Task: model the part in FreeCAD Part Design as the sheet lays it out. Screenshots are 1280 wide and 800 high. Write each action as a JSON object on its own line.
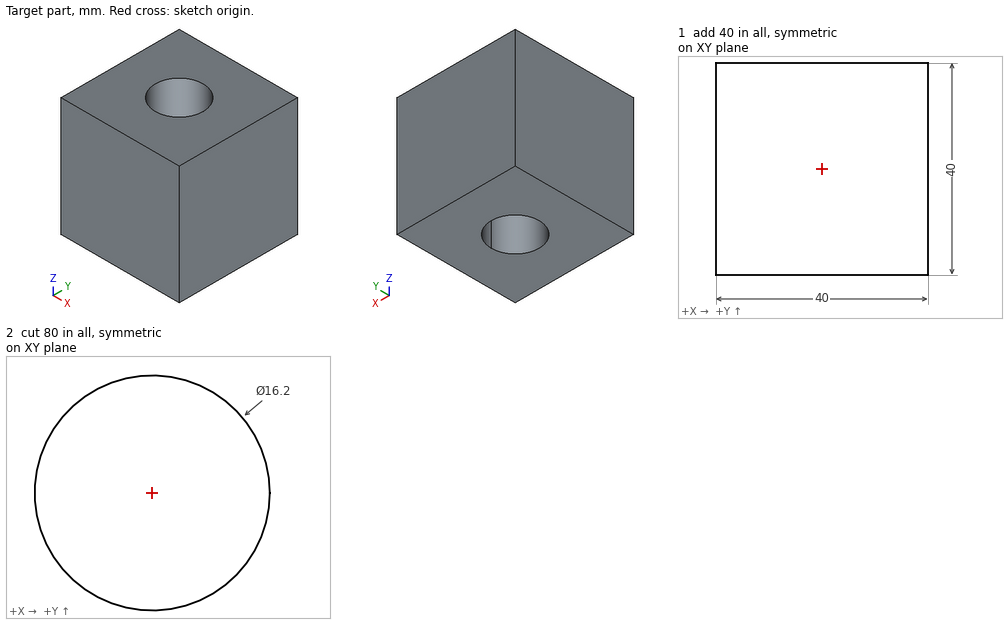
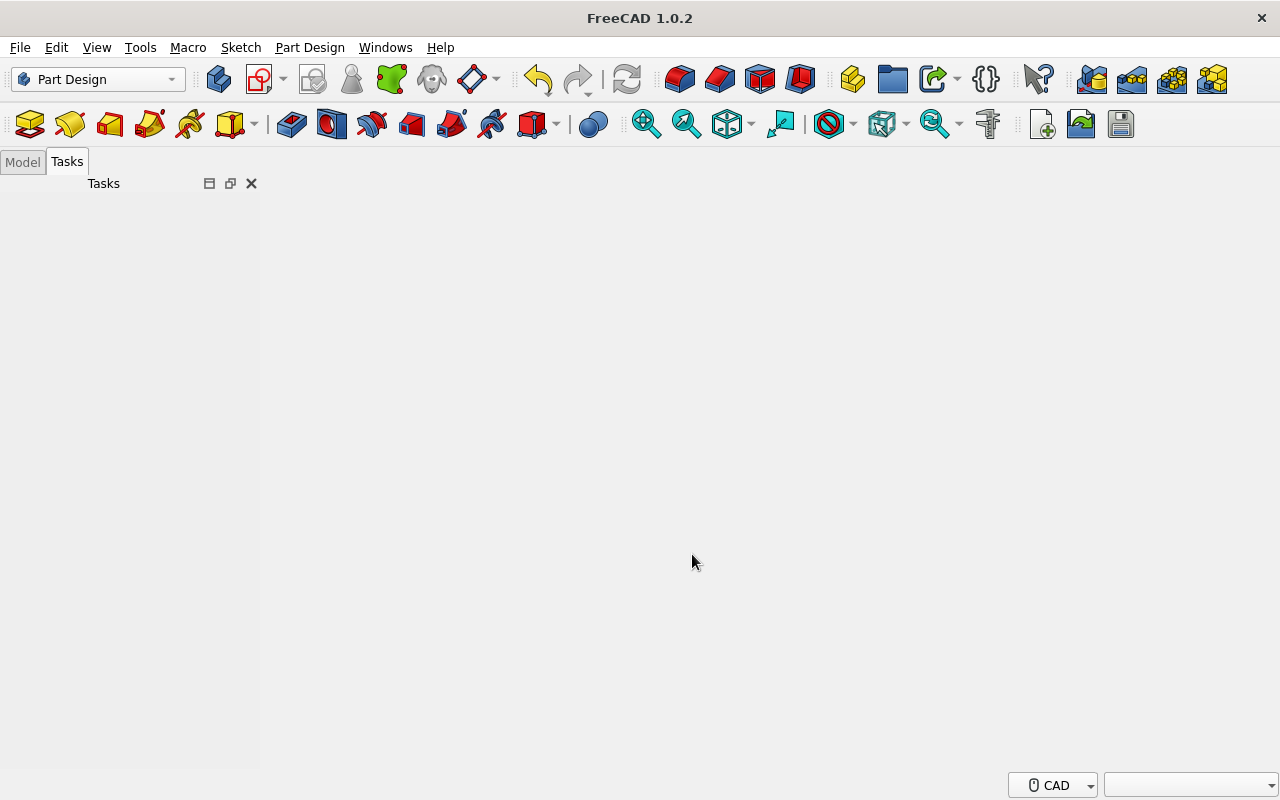
{"action": "left_click", "coordinate": [1042, 124]}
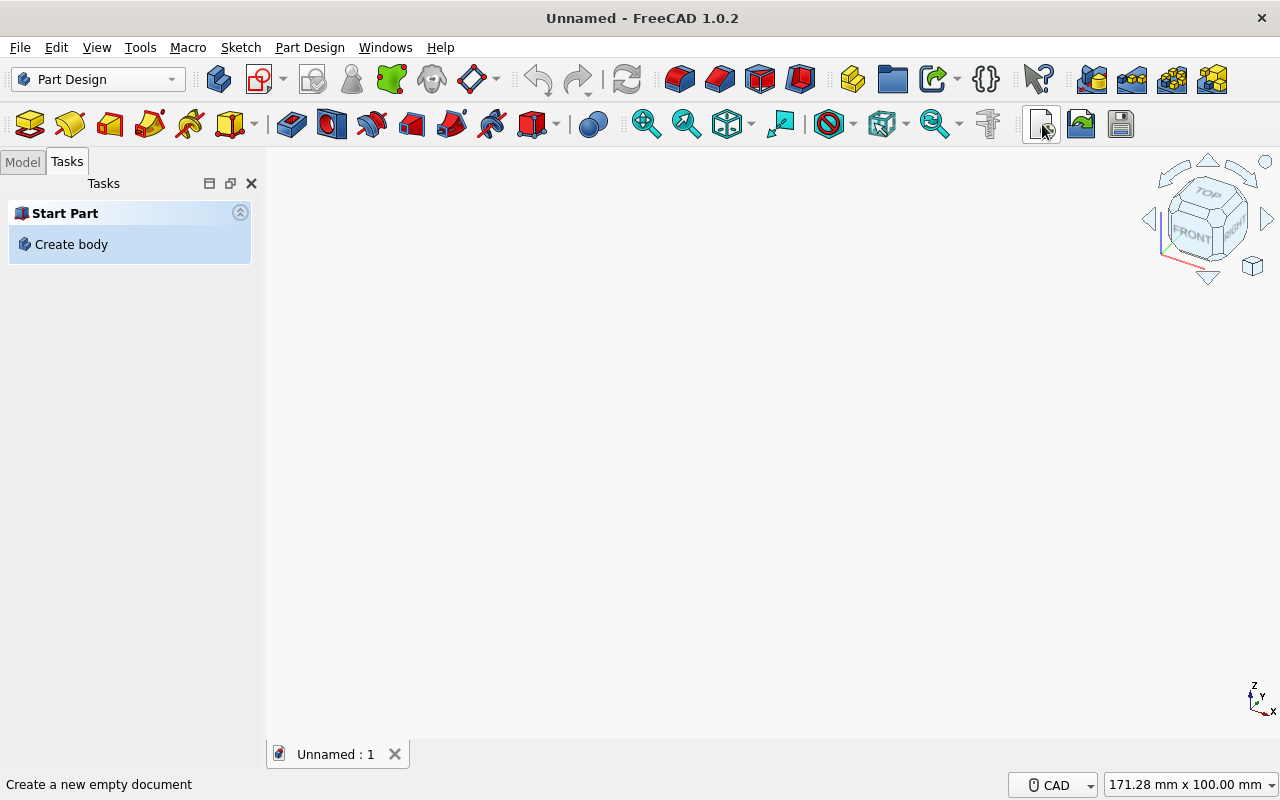
{"action": "left_click", "coordinate": [260, 80]}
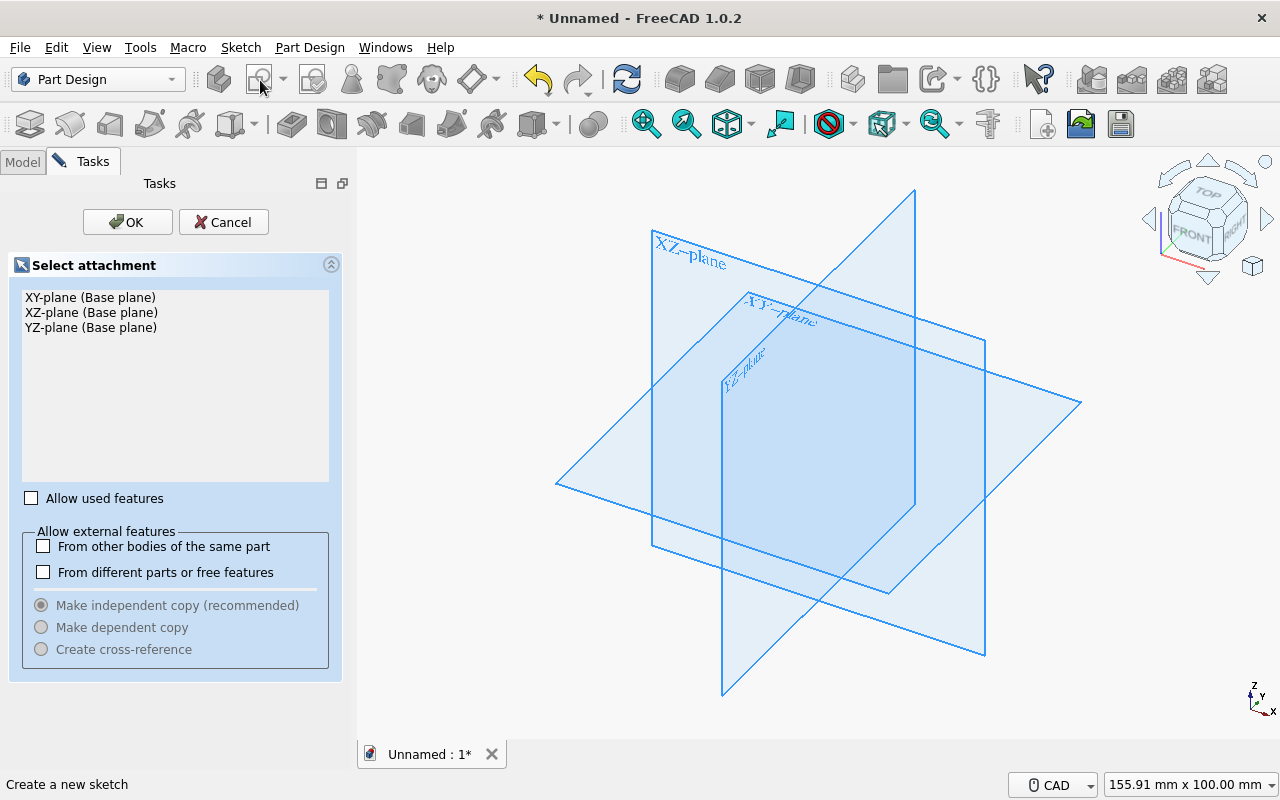
{"action": "left_click", "coordinate": [82, 298]}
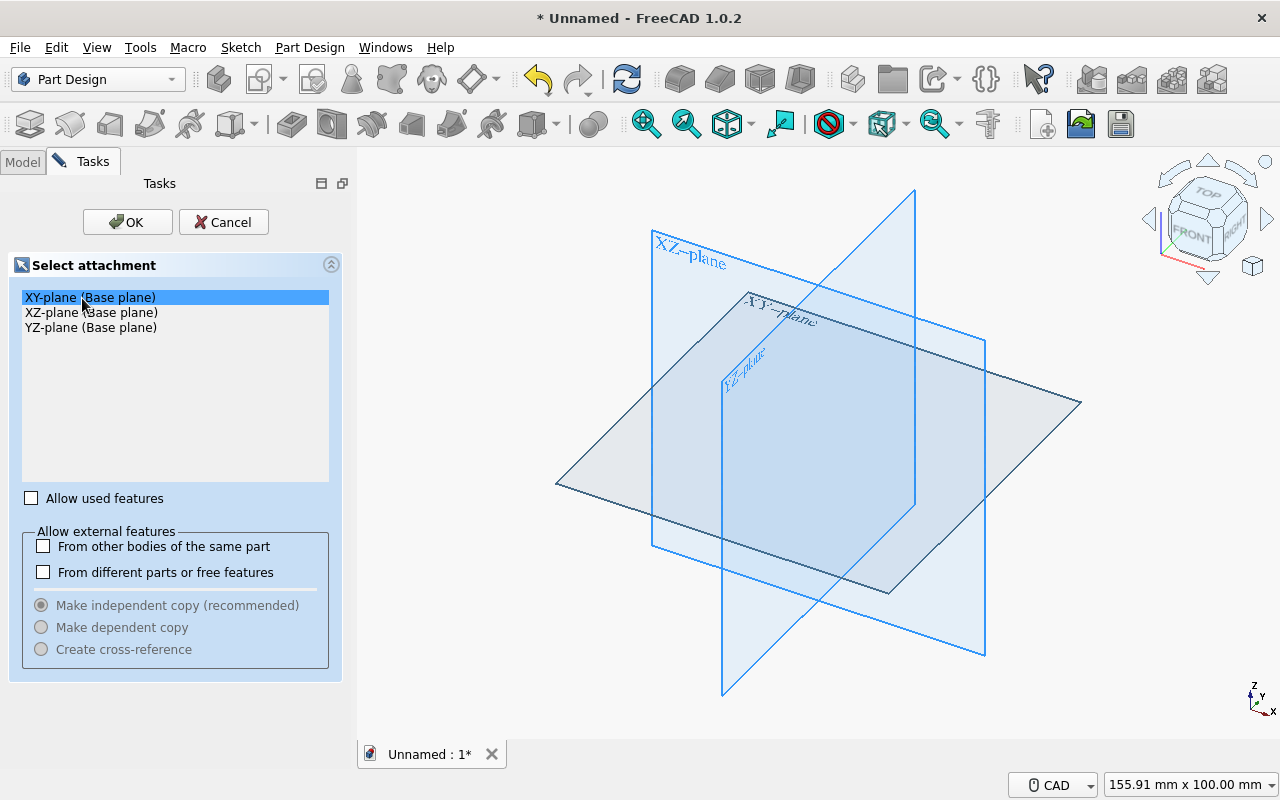
{"action": "left_click", "coordinate": [128, 222]}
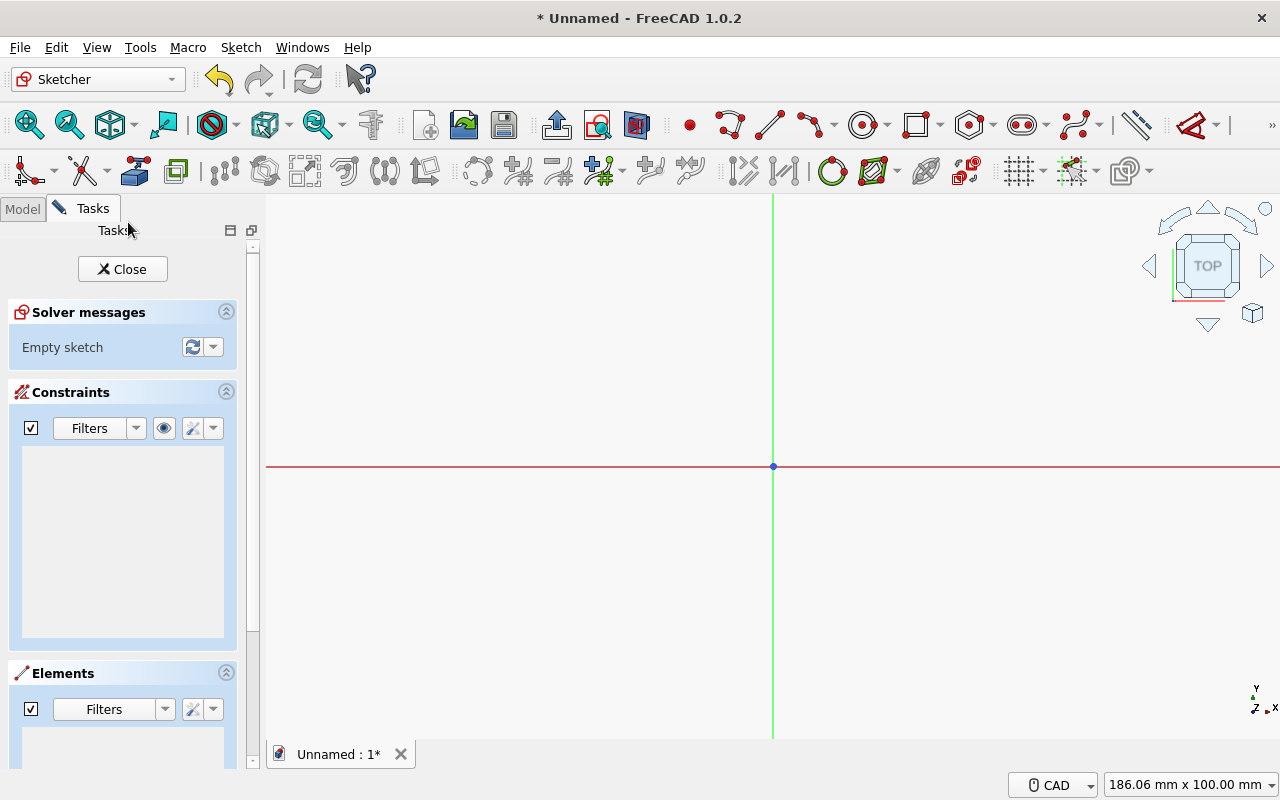
{"action": "scroll", "coordinate": [912, 467], "scroll_direction": "up", "scroll_amount": 2}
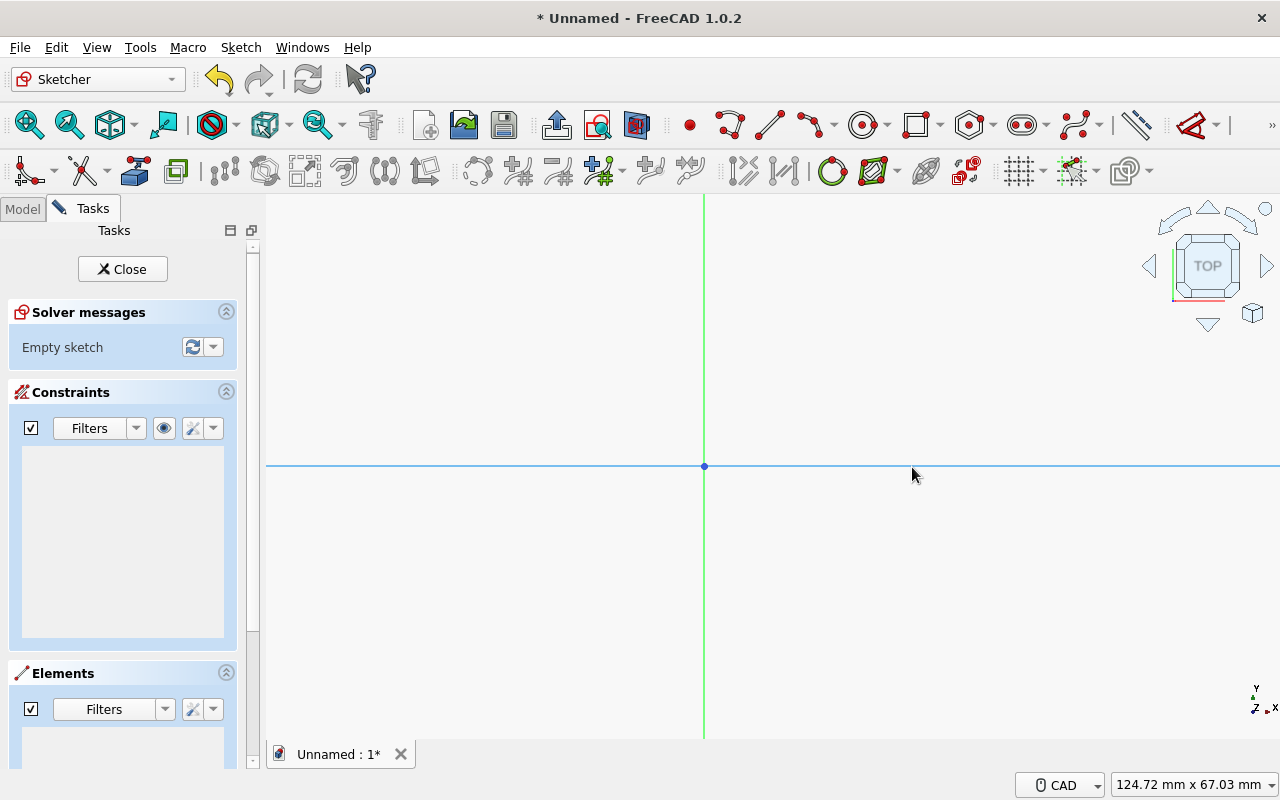
{"action": "key", "text": "g v"}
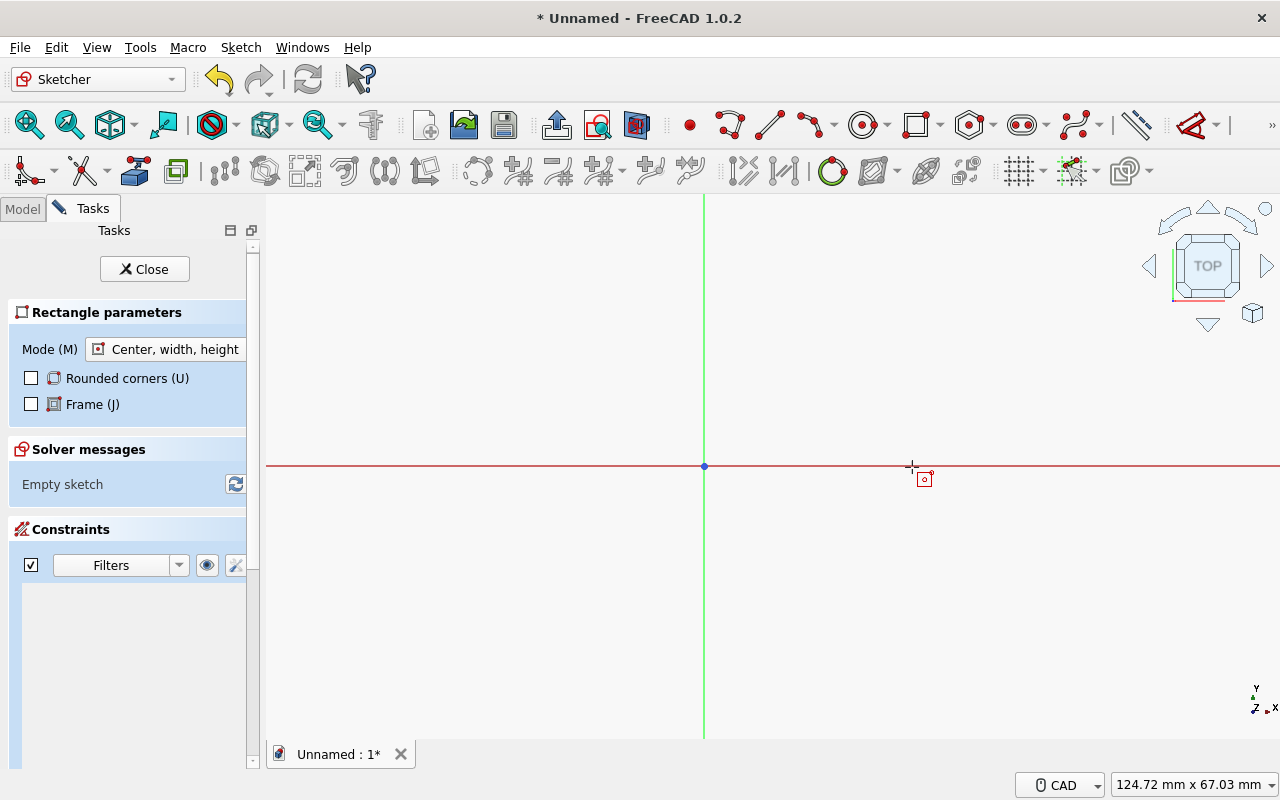
{"action": "left_click", "coordinate": [704, 466]}
{"action": "mouse_move", "coordinate": [867, 303]}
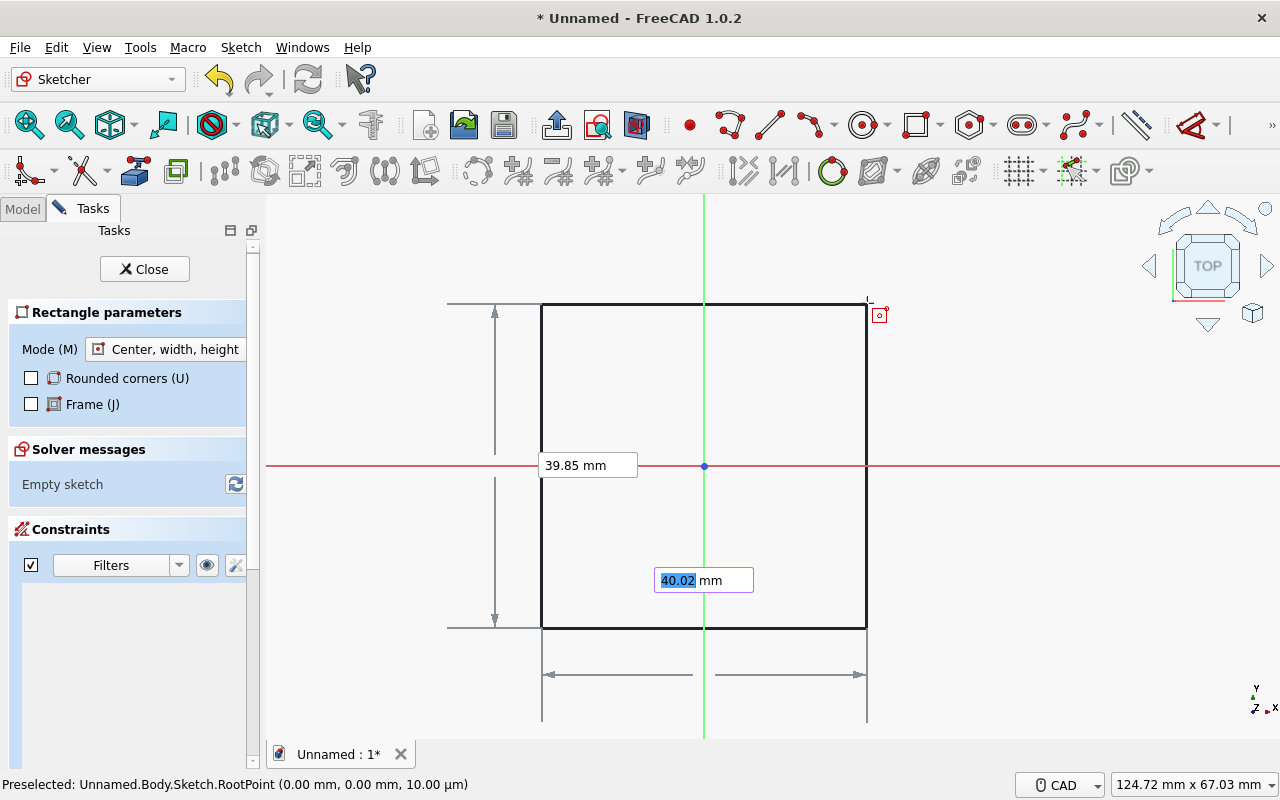
{"action": "type", "text": "40"}
{"action": "key", "text": "Tab"}
{"action": "type", "text": "40"}
{"action": "key", "text": "Return"}
{"action": "key", "text": "Escape"}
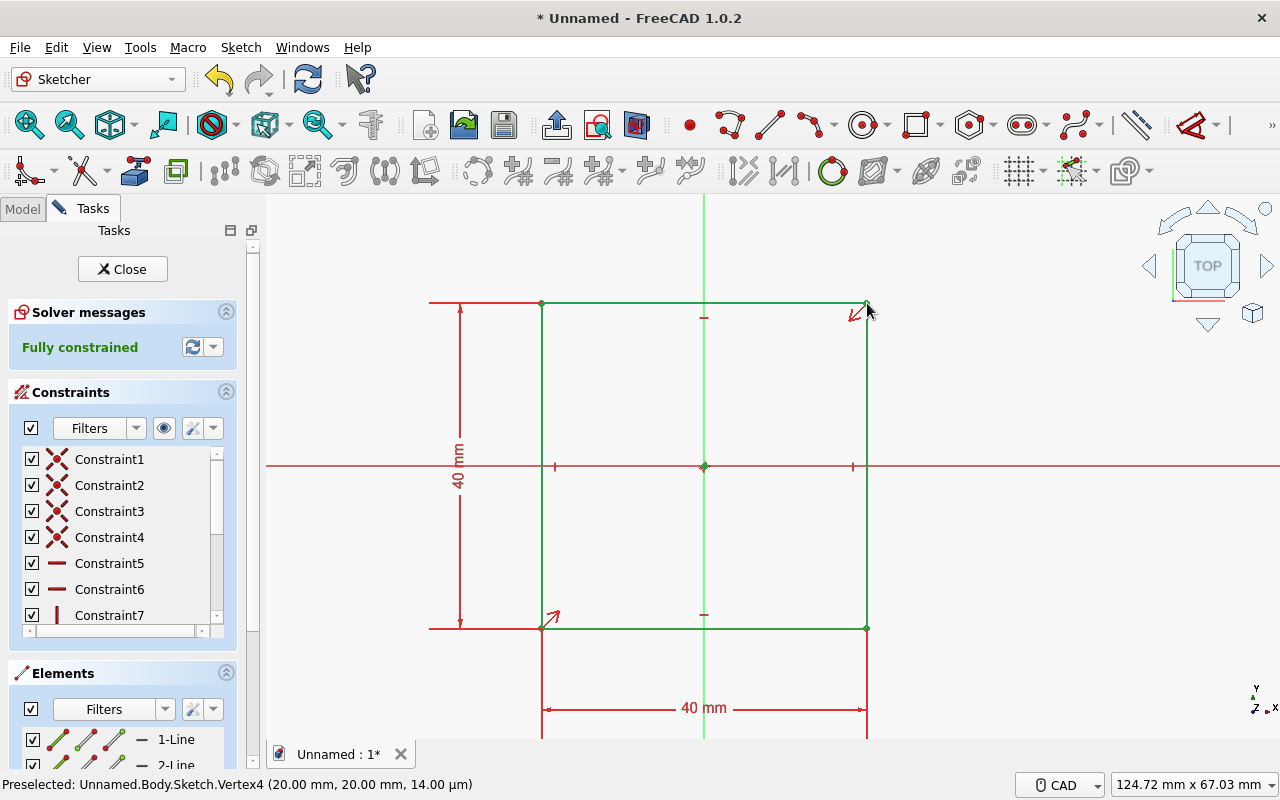
{"action": "left_click", "coordinate": [123, 269]}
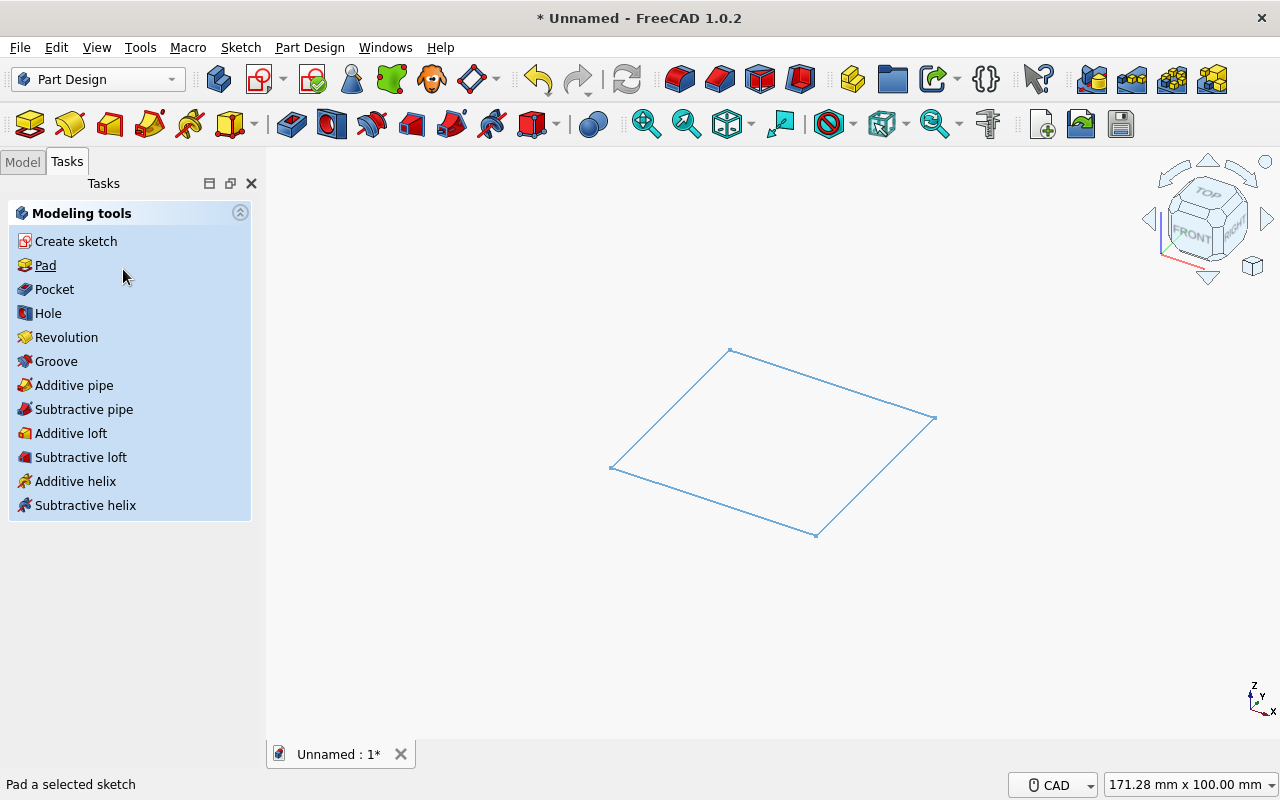
{"action": "left_click", "coordinate": [30, 124]}